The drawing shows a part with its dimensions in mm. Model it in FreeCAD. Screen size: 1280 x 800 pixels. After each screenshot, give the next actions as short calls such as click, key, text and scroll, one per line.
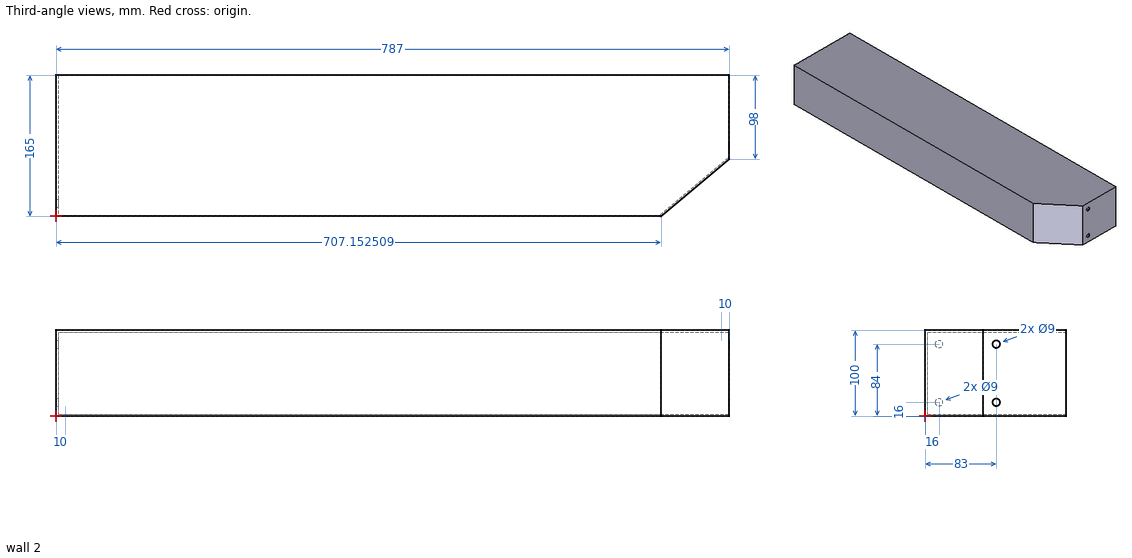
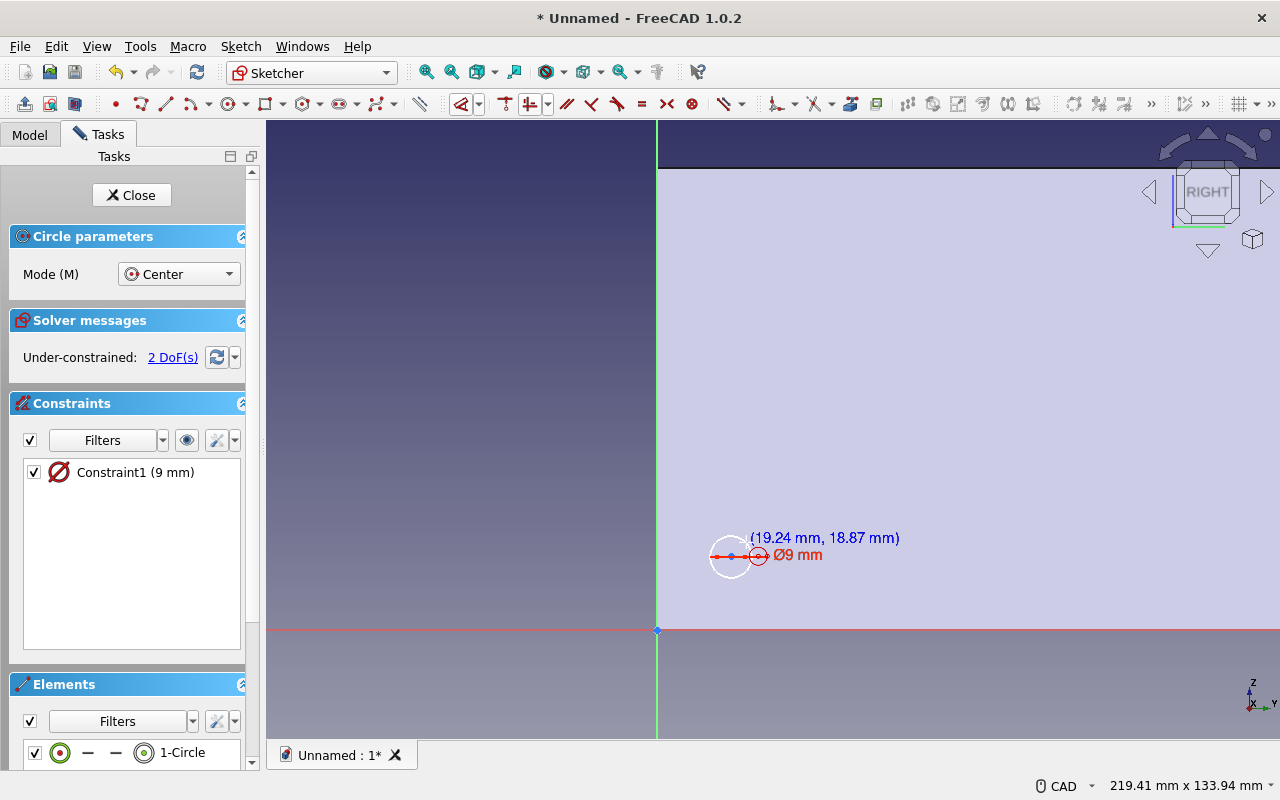
click(731, 242)
move(746, 227)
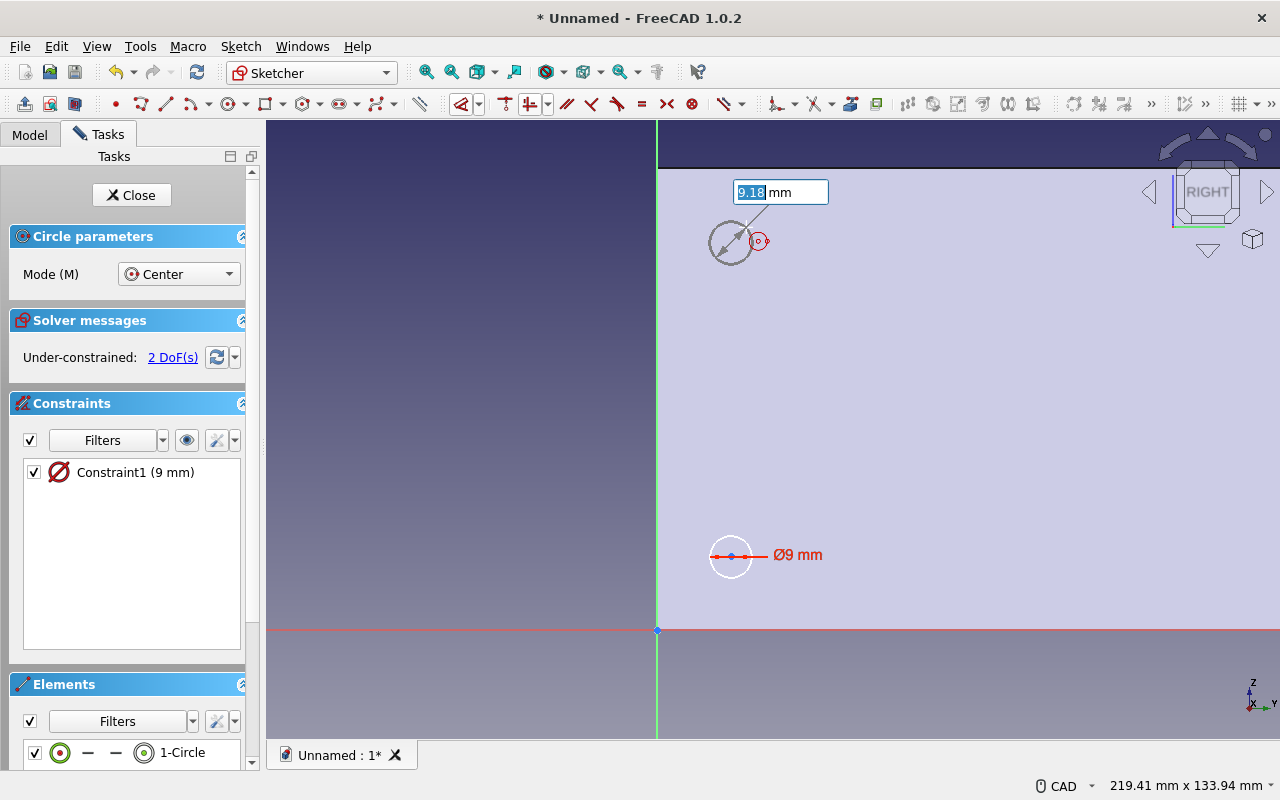
text(9)
key(Return)
key(Escape)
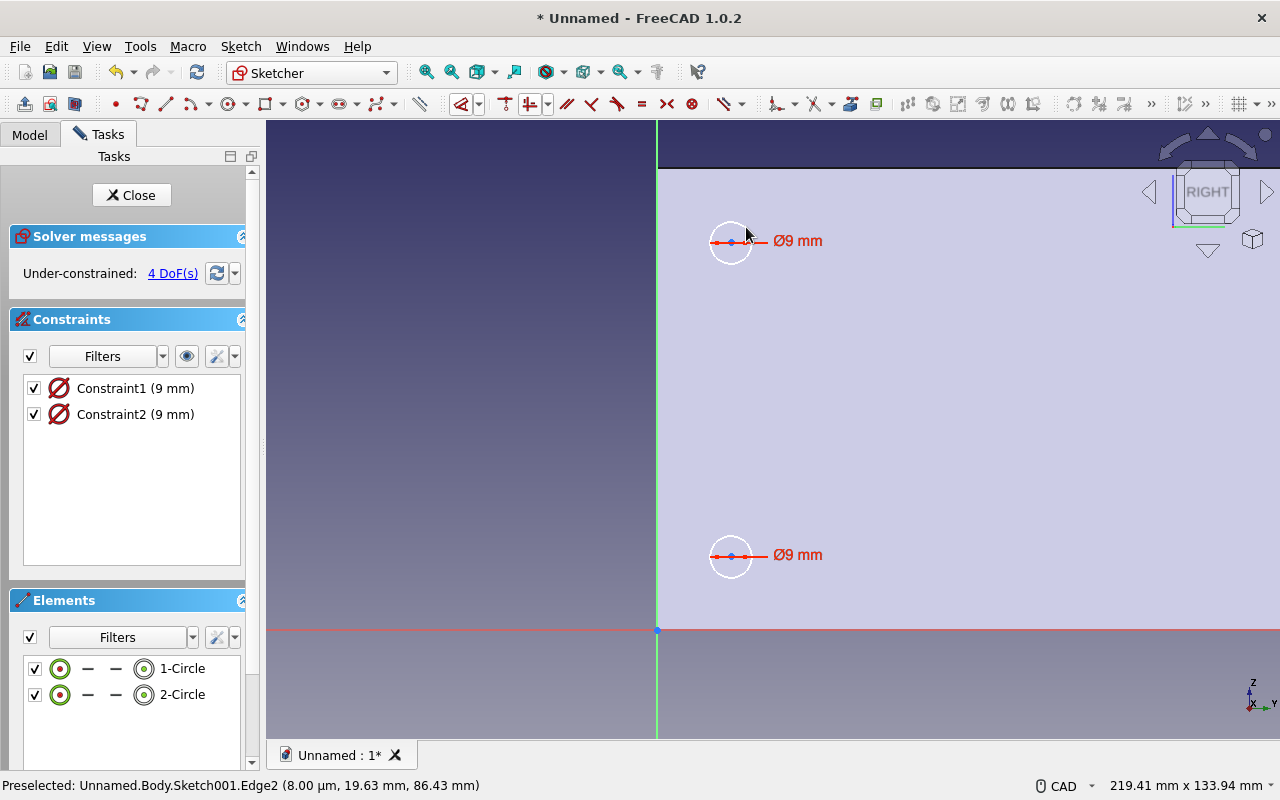
click(731, 557)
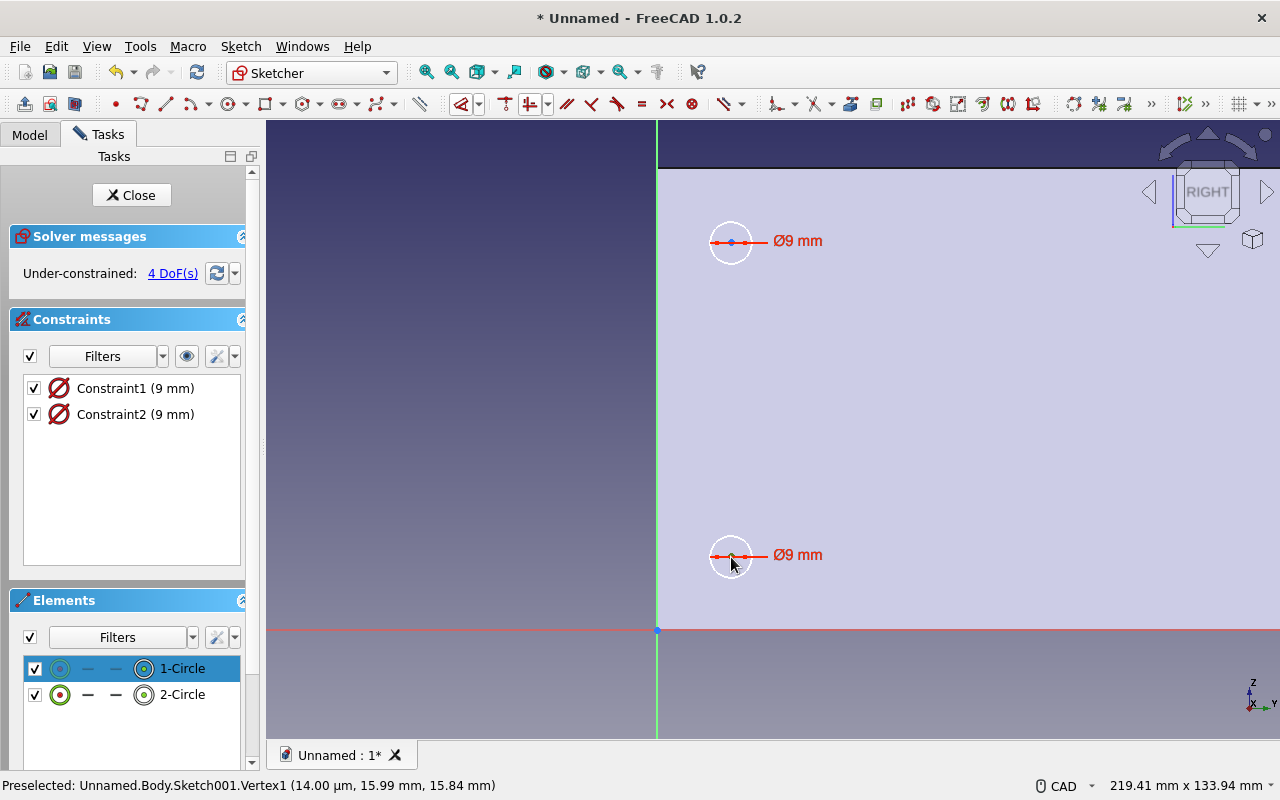
click(731, 243)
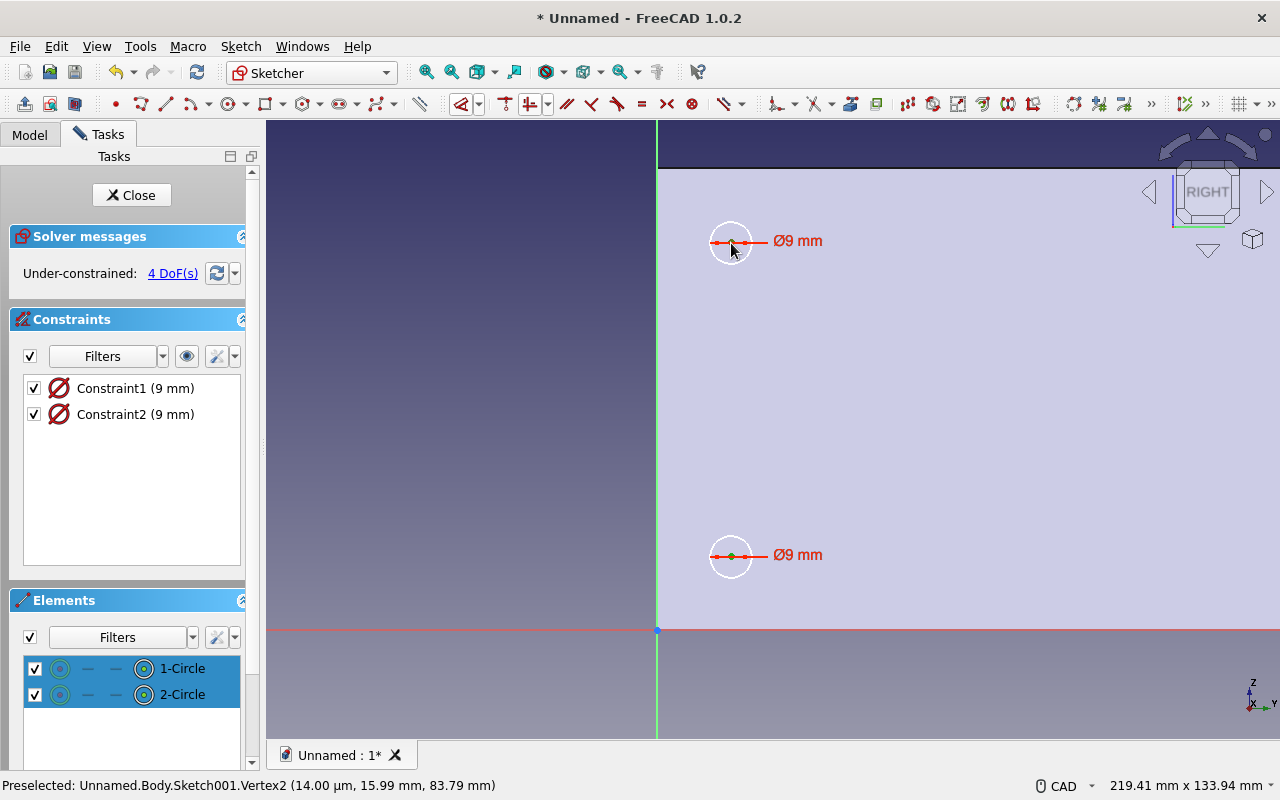
click(548, 104)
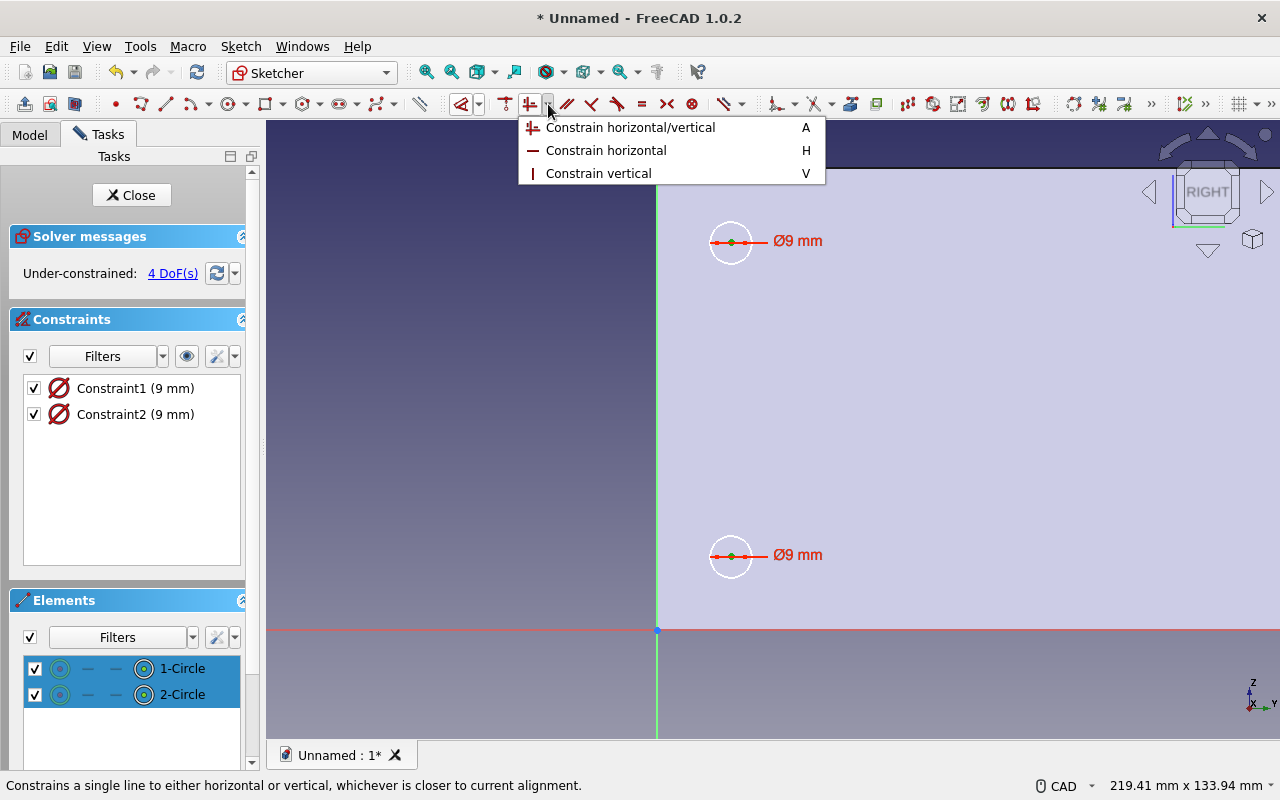
click(672, 174)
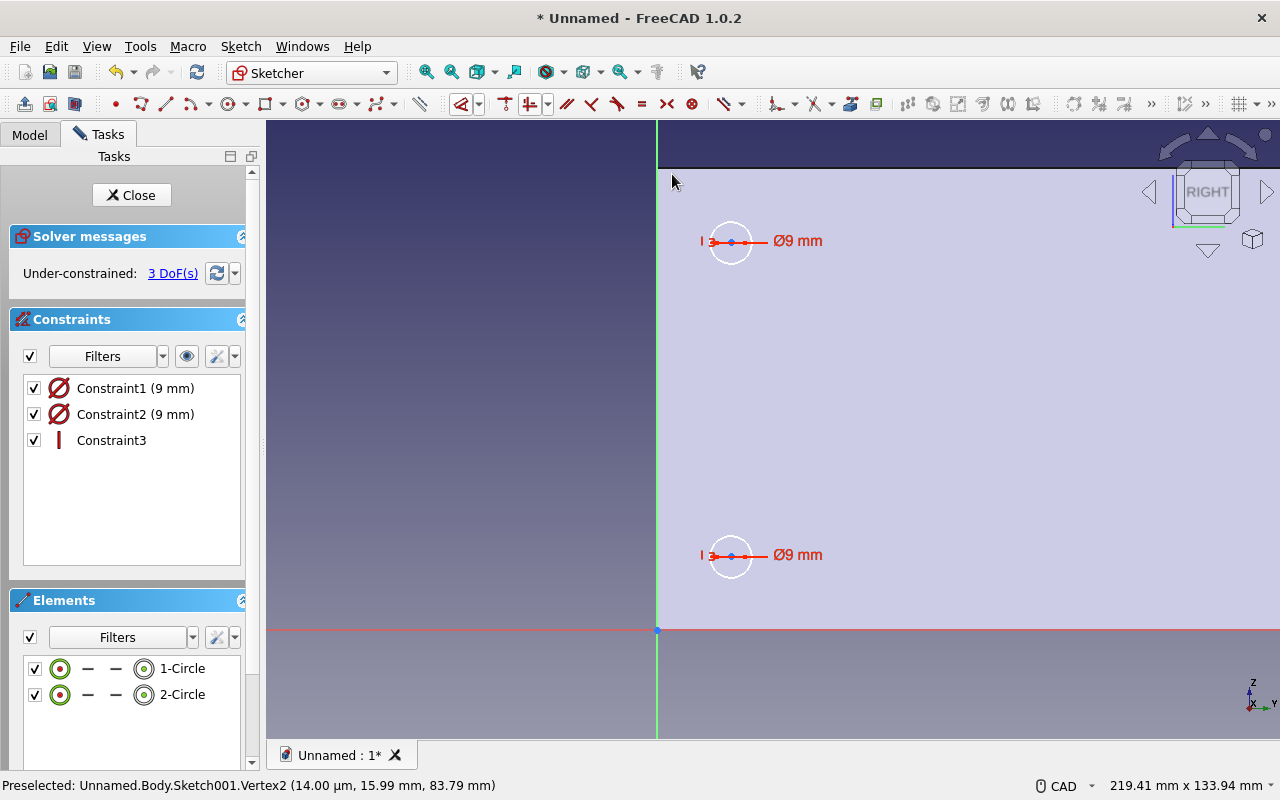
click(731, 557)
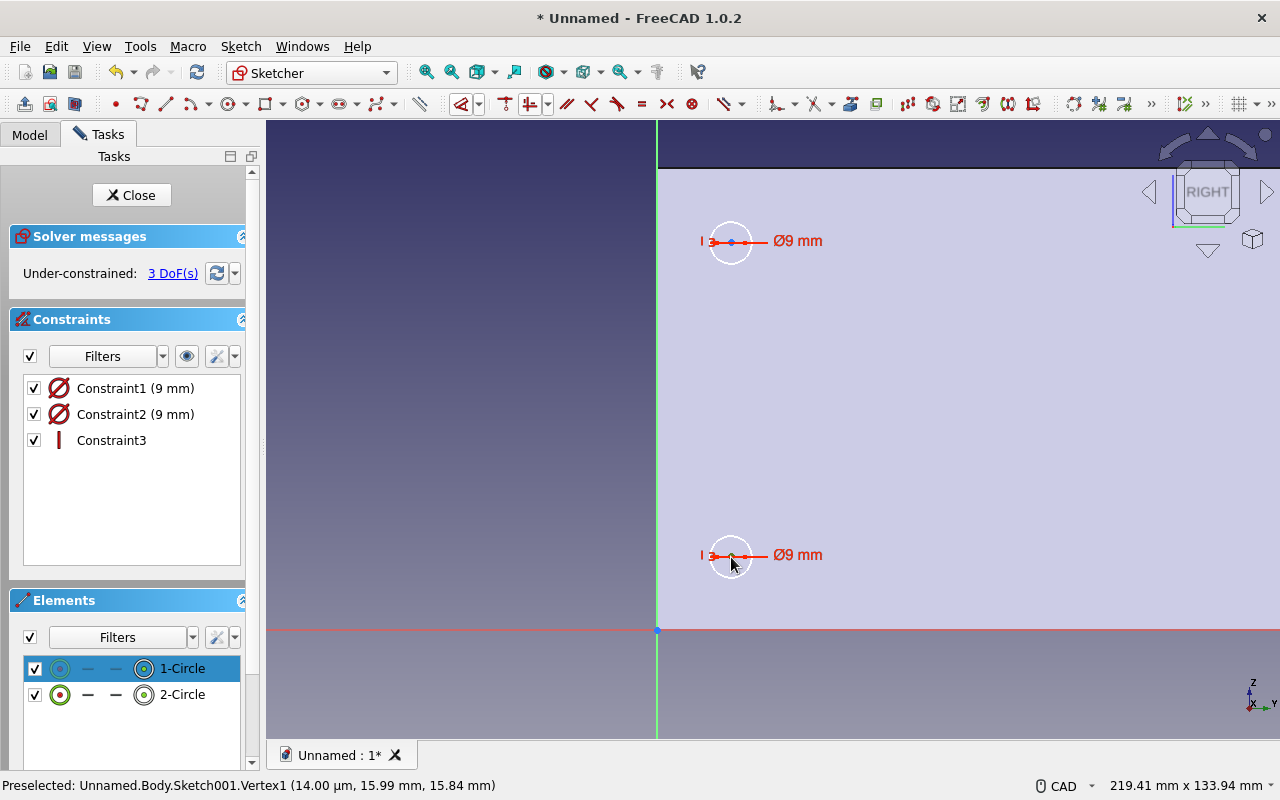
click(478, 104)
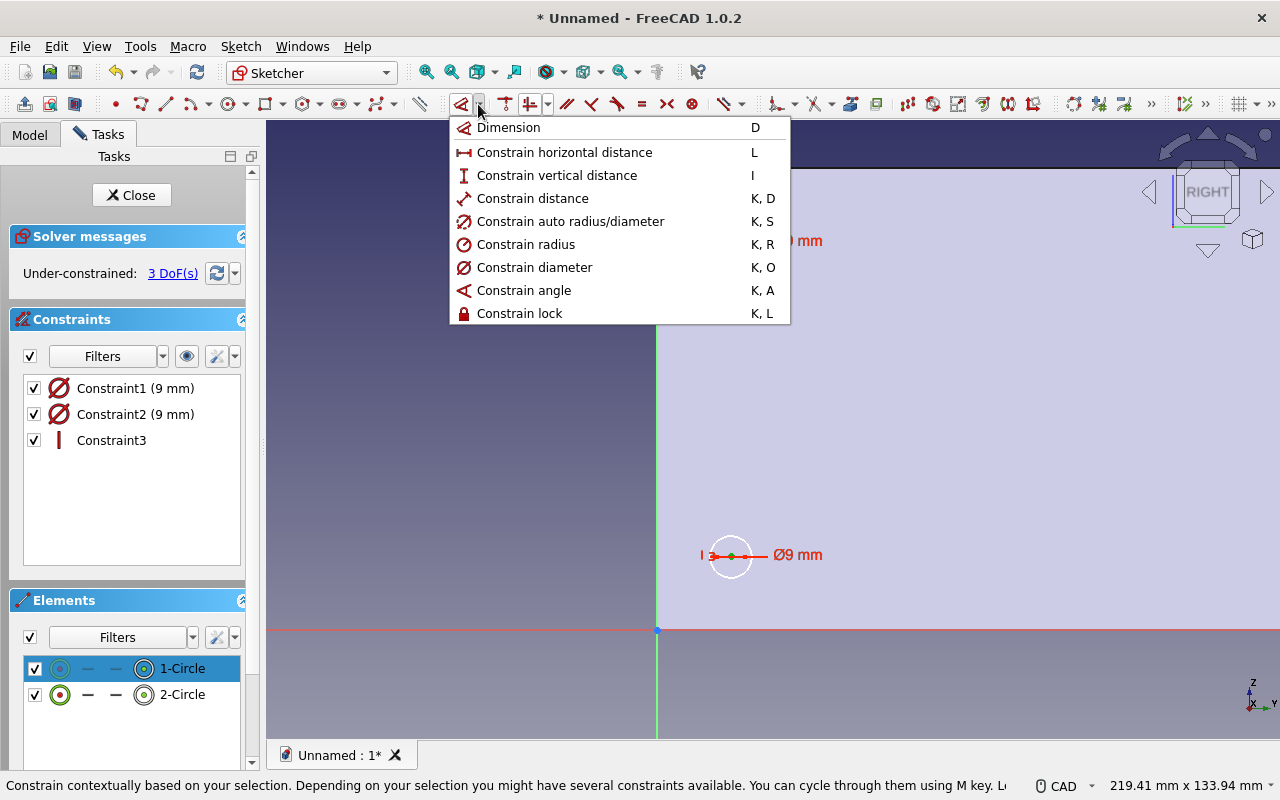
click(620, 152)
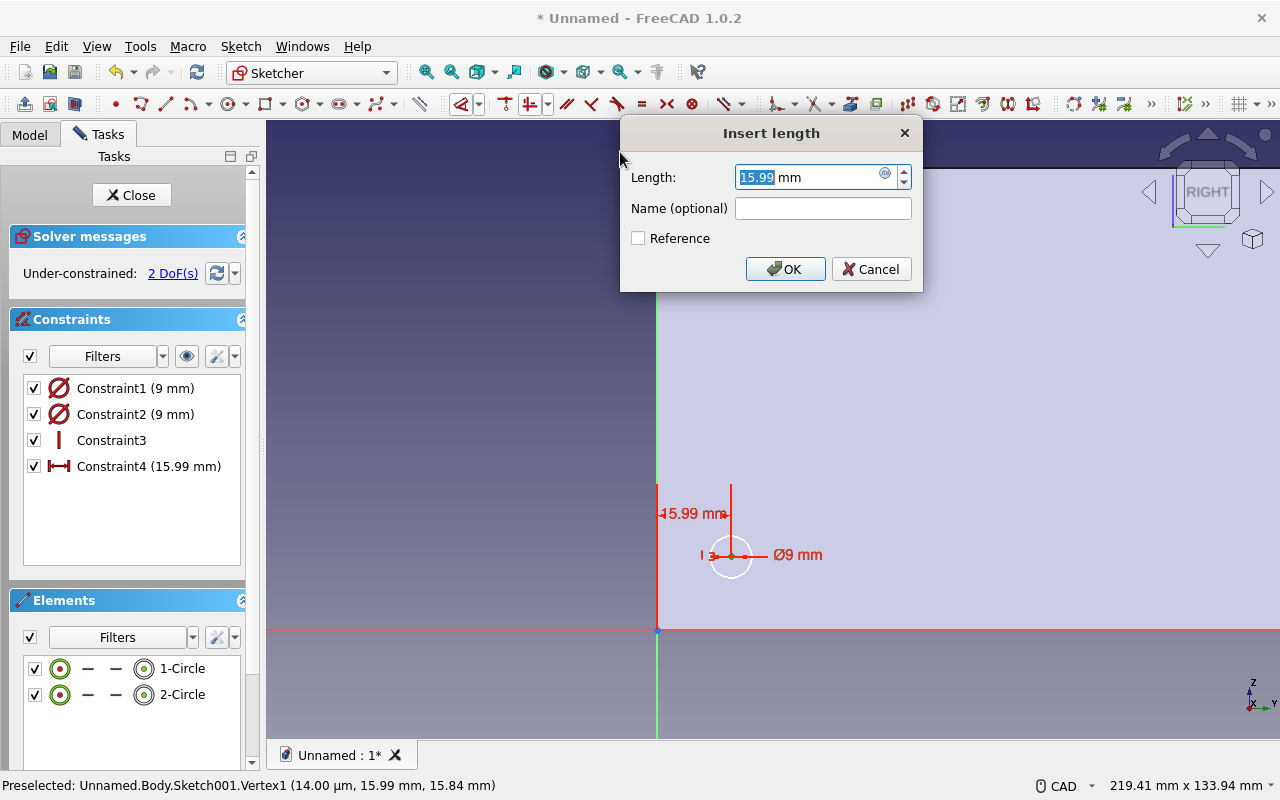
text(16)
key(Return)